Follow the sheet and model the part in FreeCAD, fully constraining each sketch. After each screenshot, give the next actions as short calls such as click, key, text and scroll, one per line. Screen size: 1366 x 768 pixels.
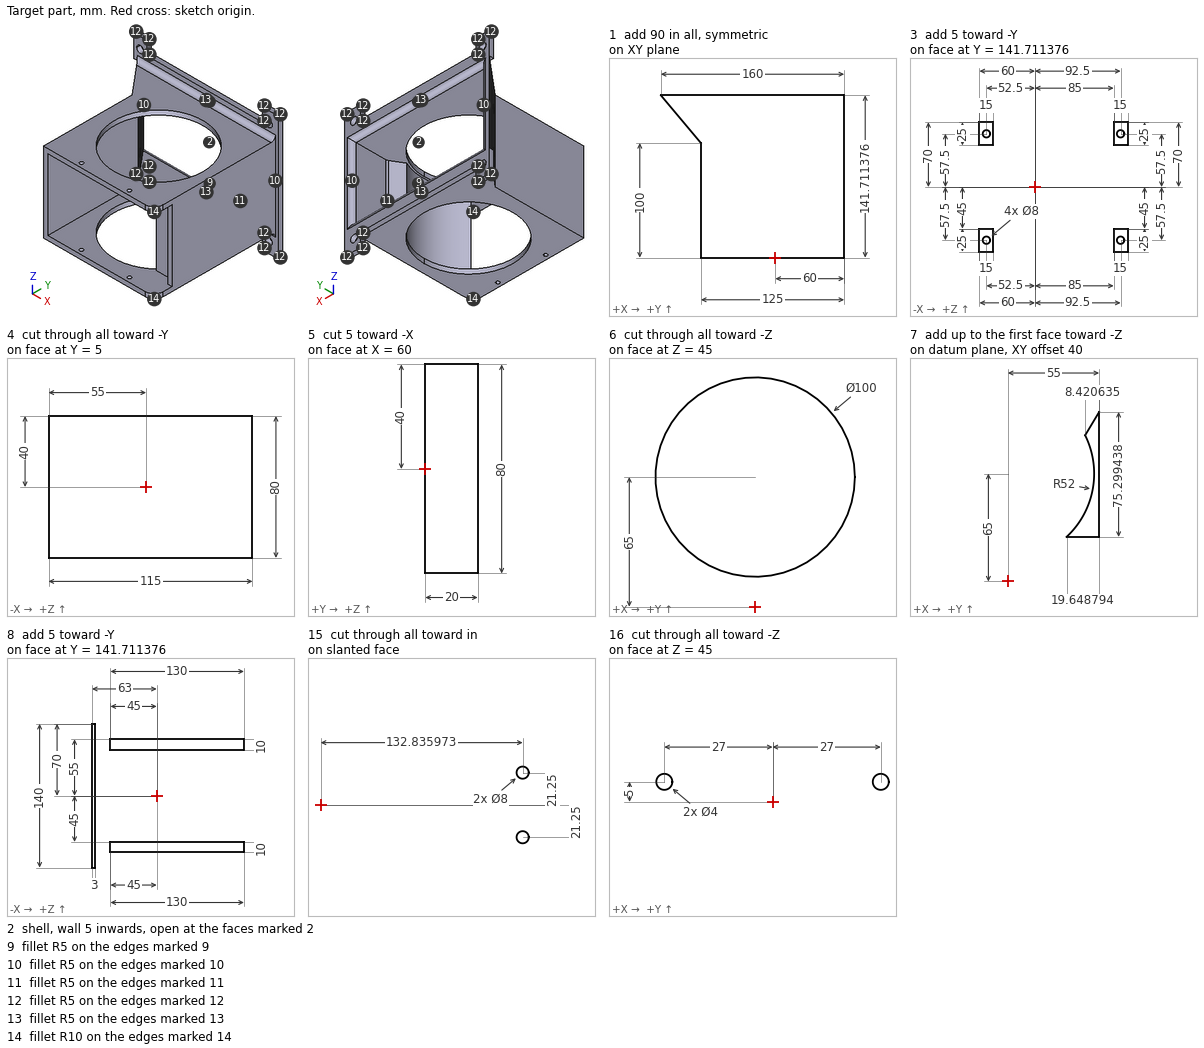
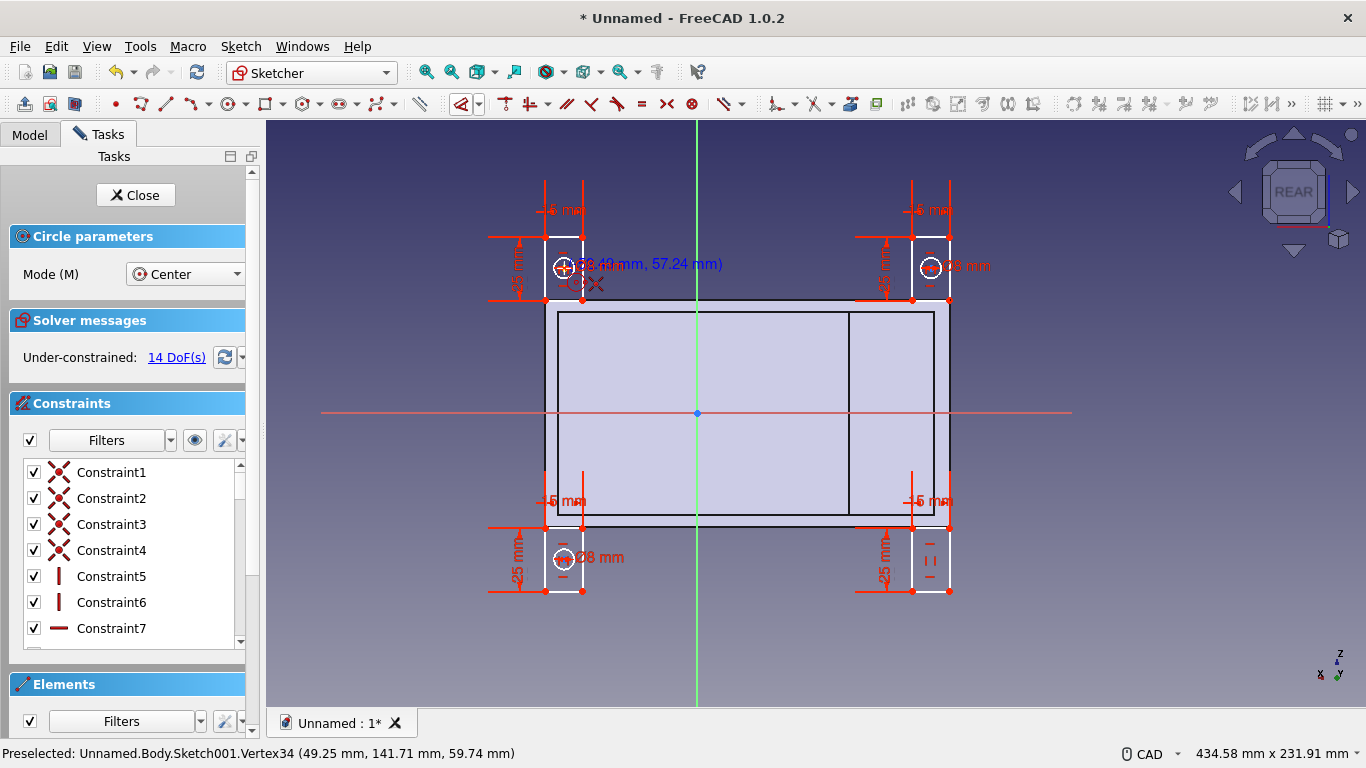
scroll(931, 559, up, 5)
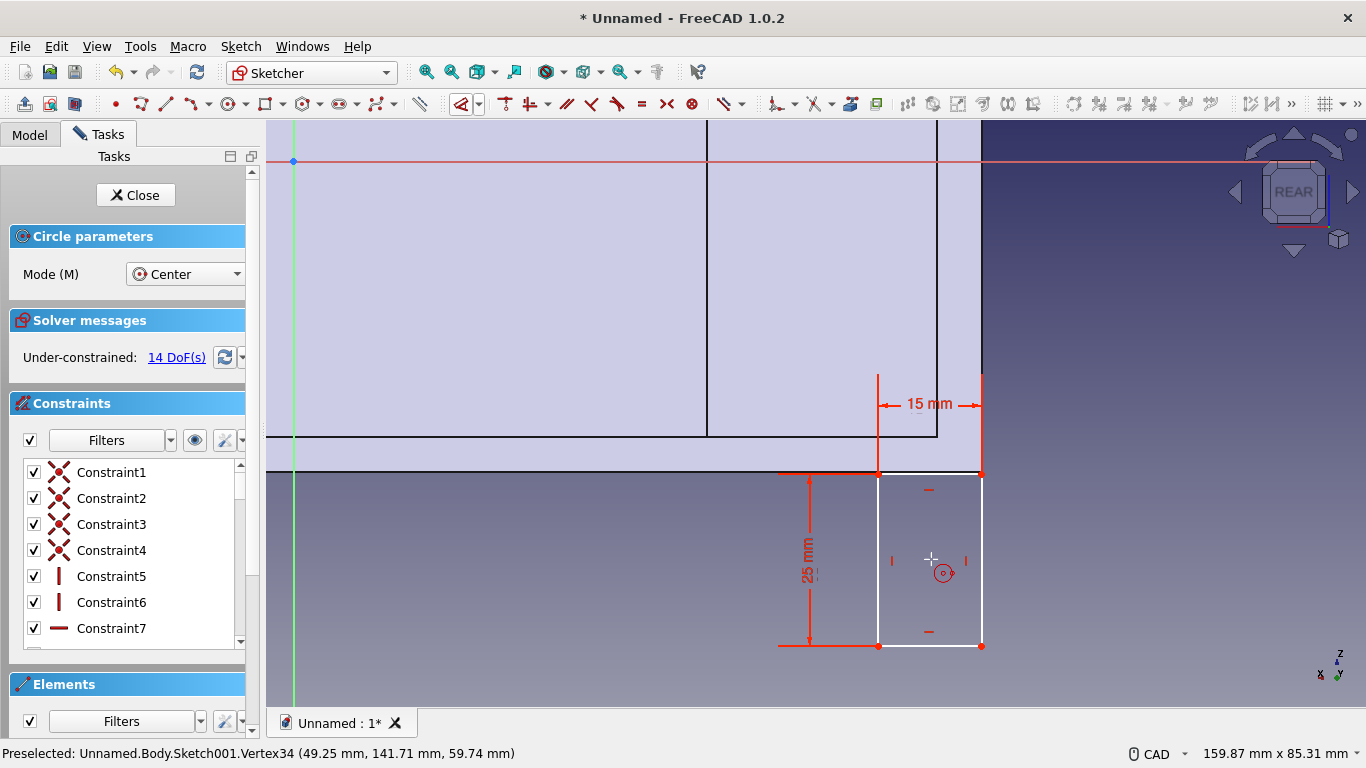
click(930, 558)
move(950, 538)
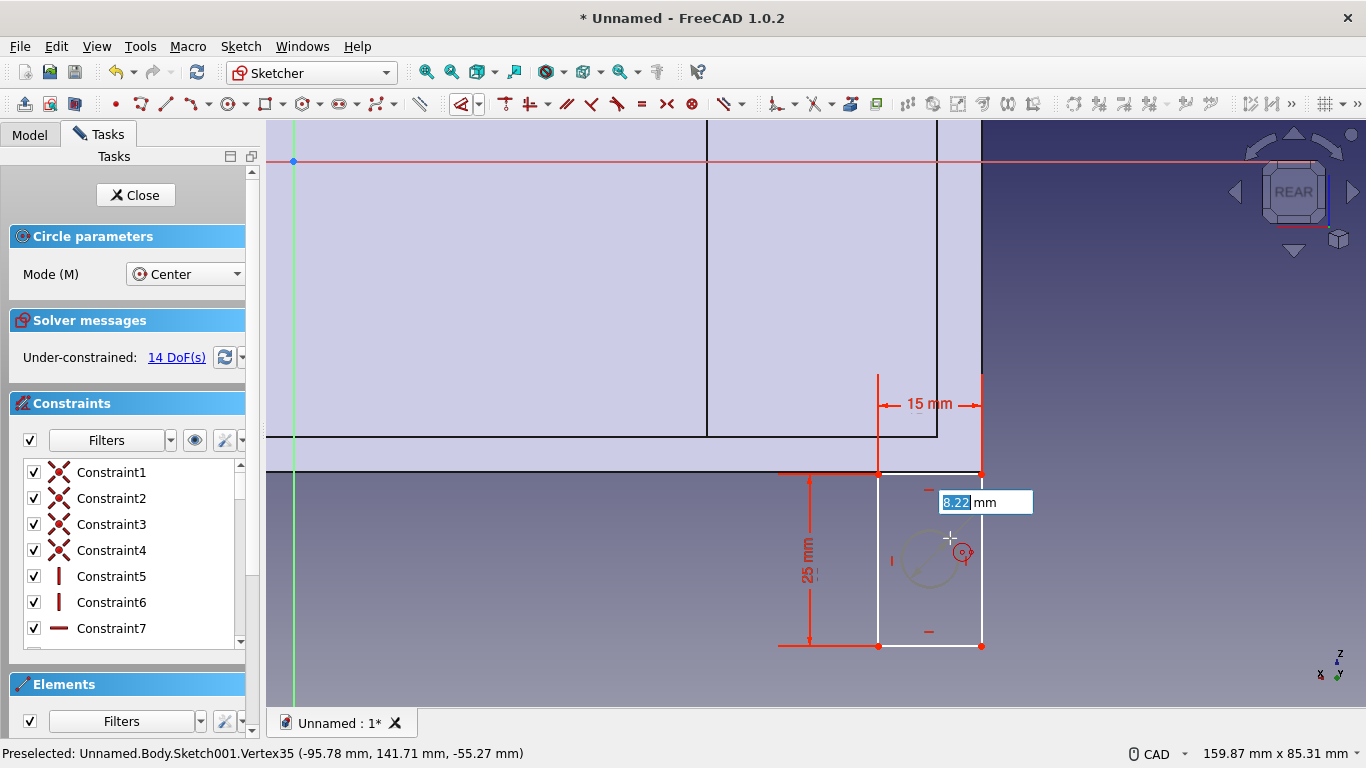
text(8)
key(Return)
key(Escape)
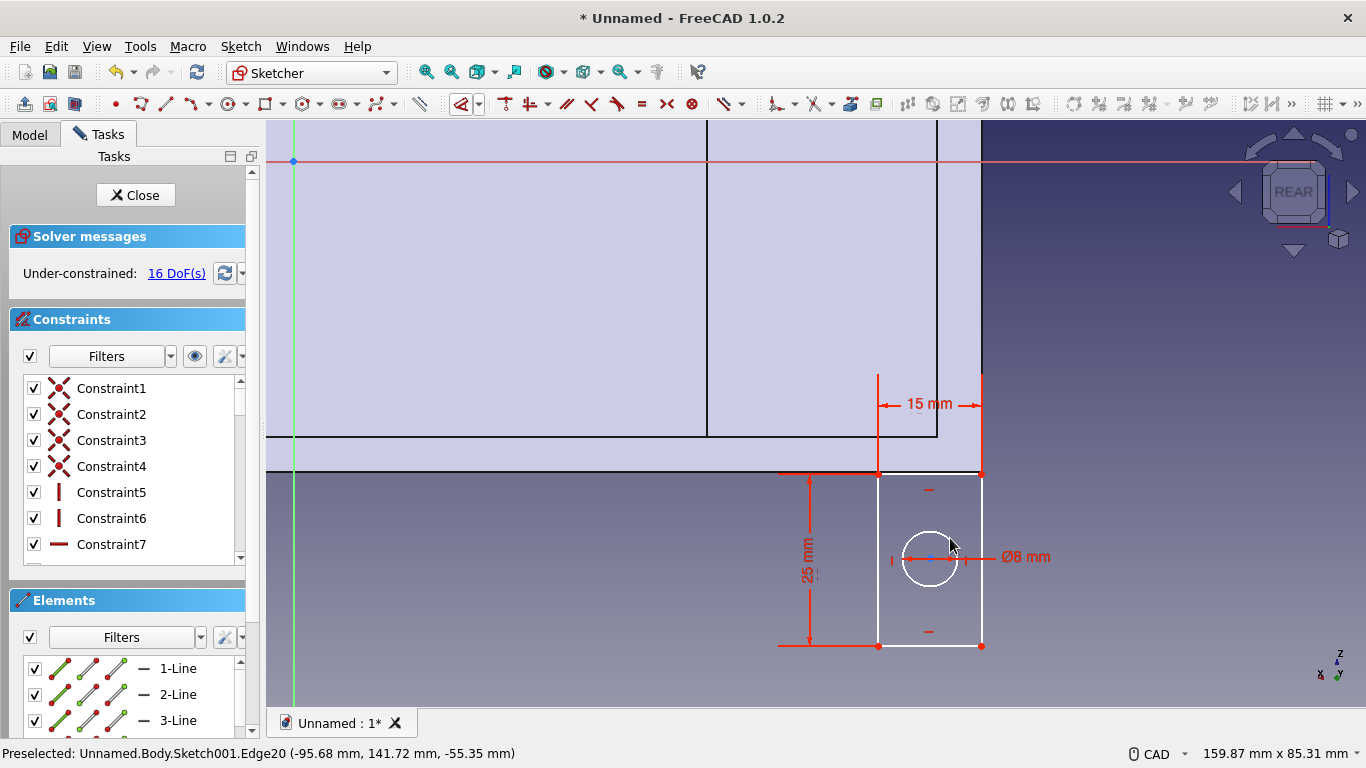
scroll(931, 560, down, 5)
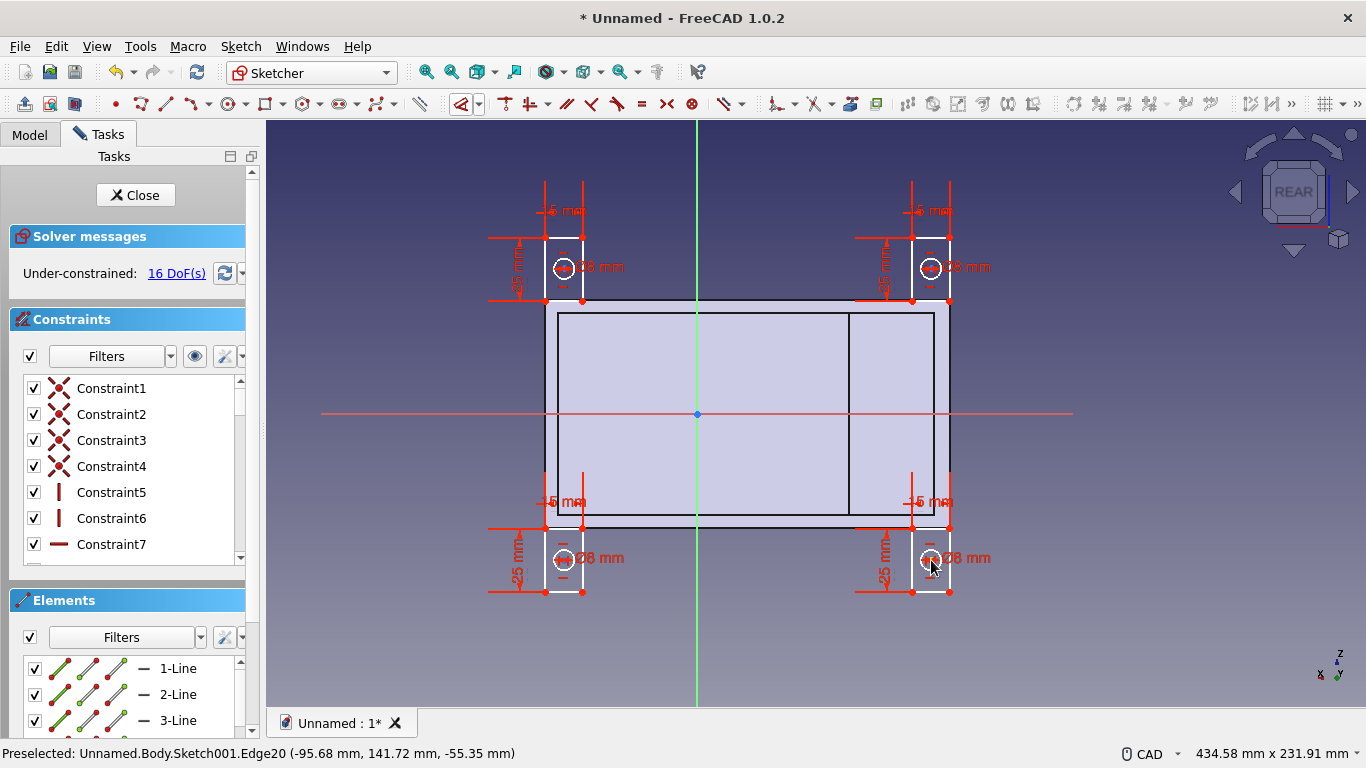
click(545, 529)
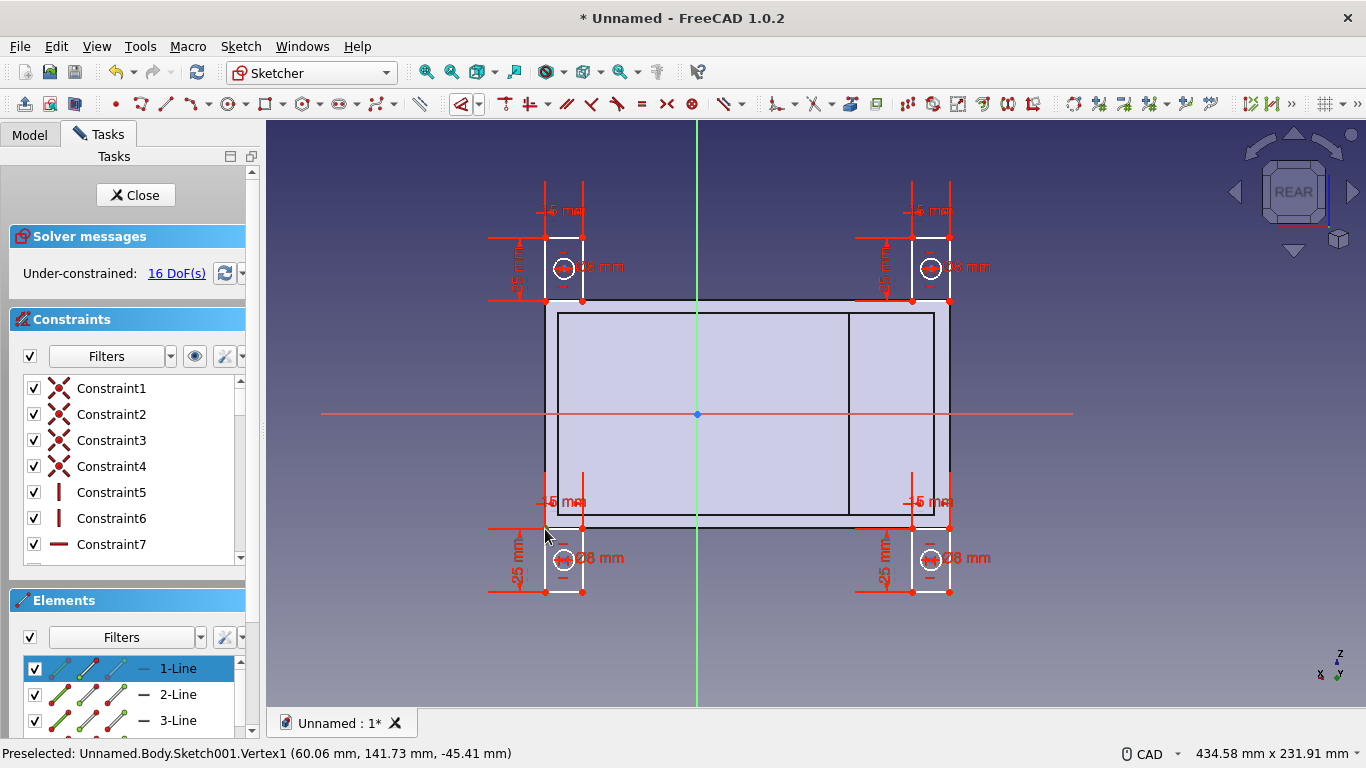
key(l)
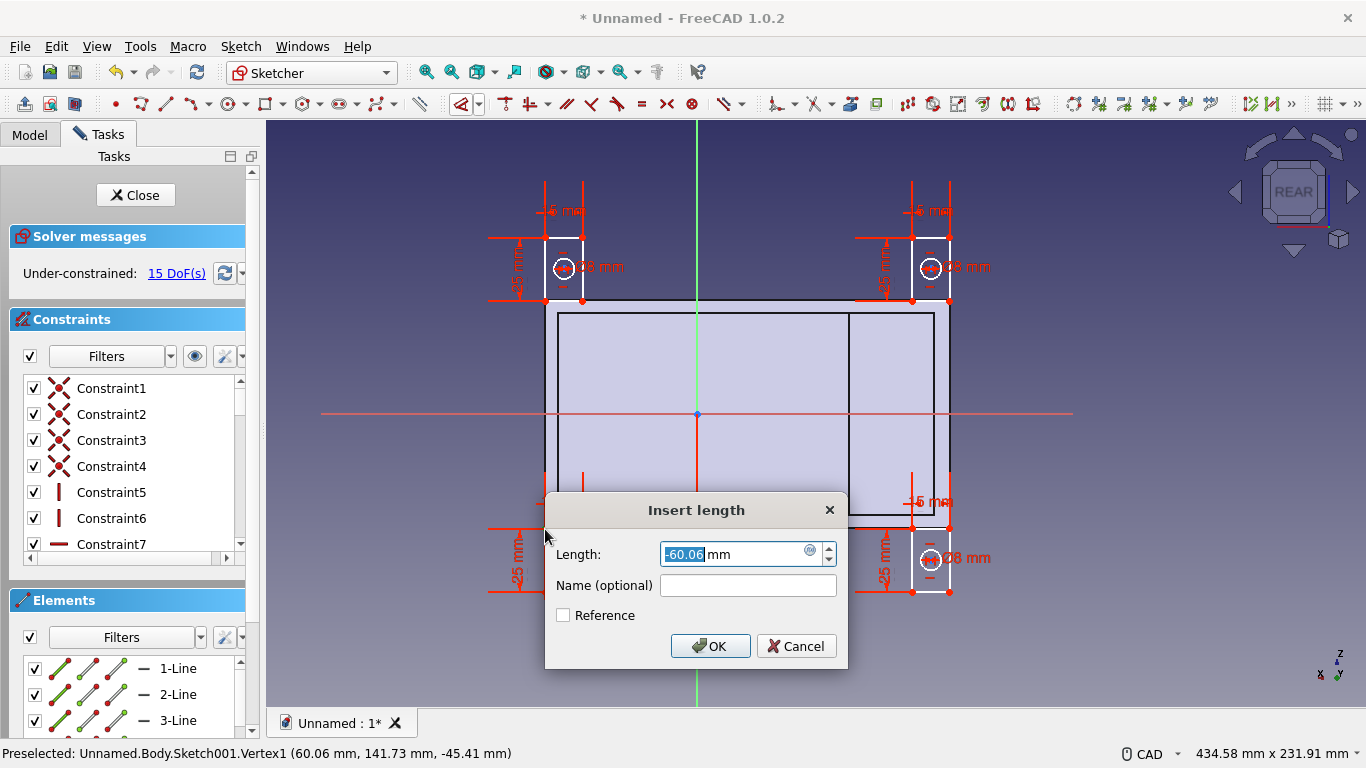
text(-60)
key(Return)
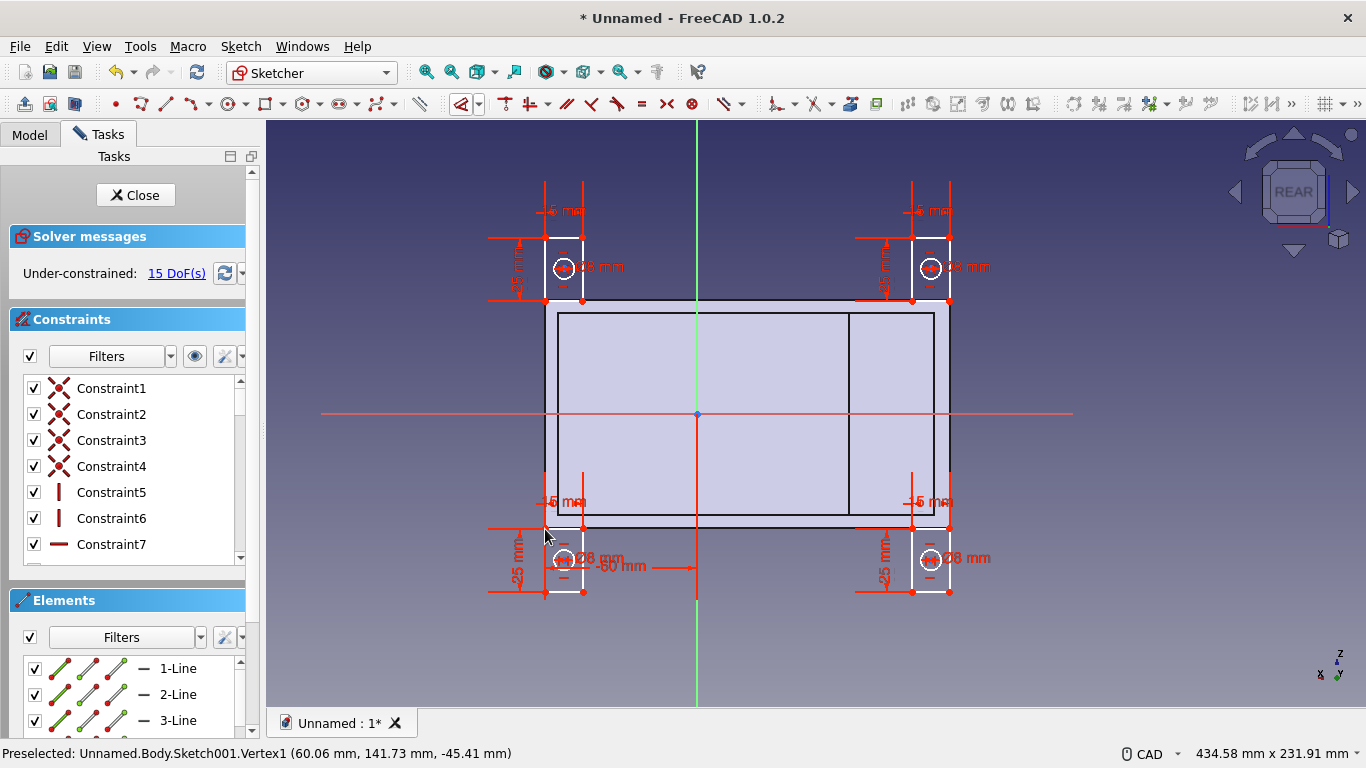
click(545, 529)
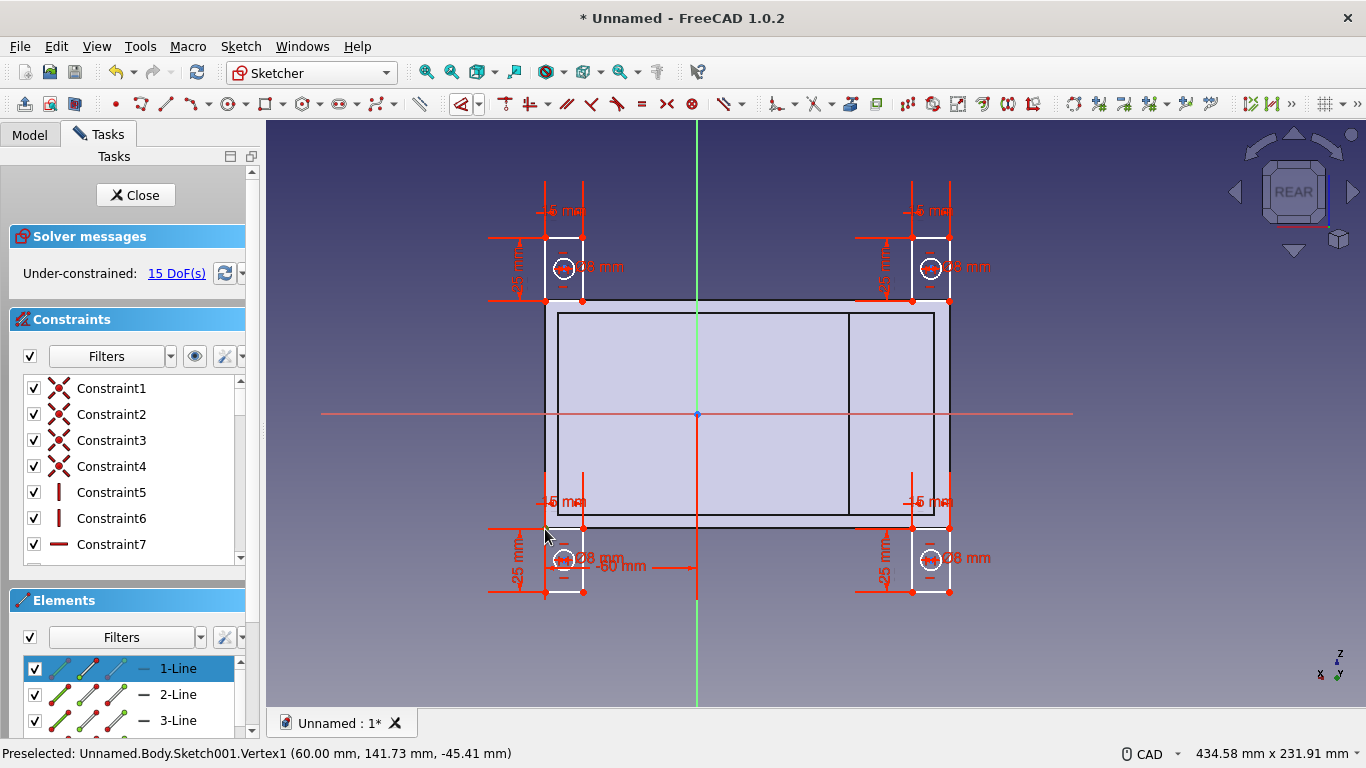
key(i)